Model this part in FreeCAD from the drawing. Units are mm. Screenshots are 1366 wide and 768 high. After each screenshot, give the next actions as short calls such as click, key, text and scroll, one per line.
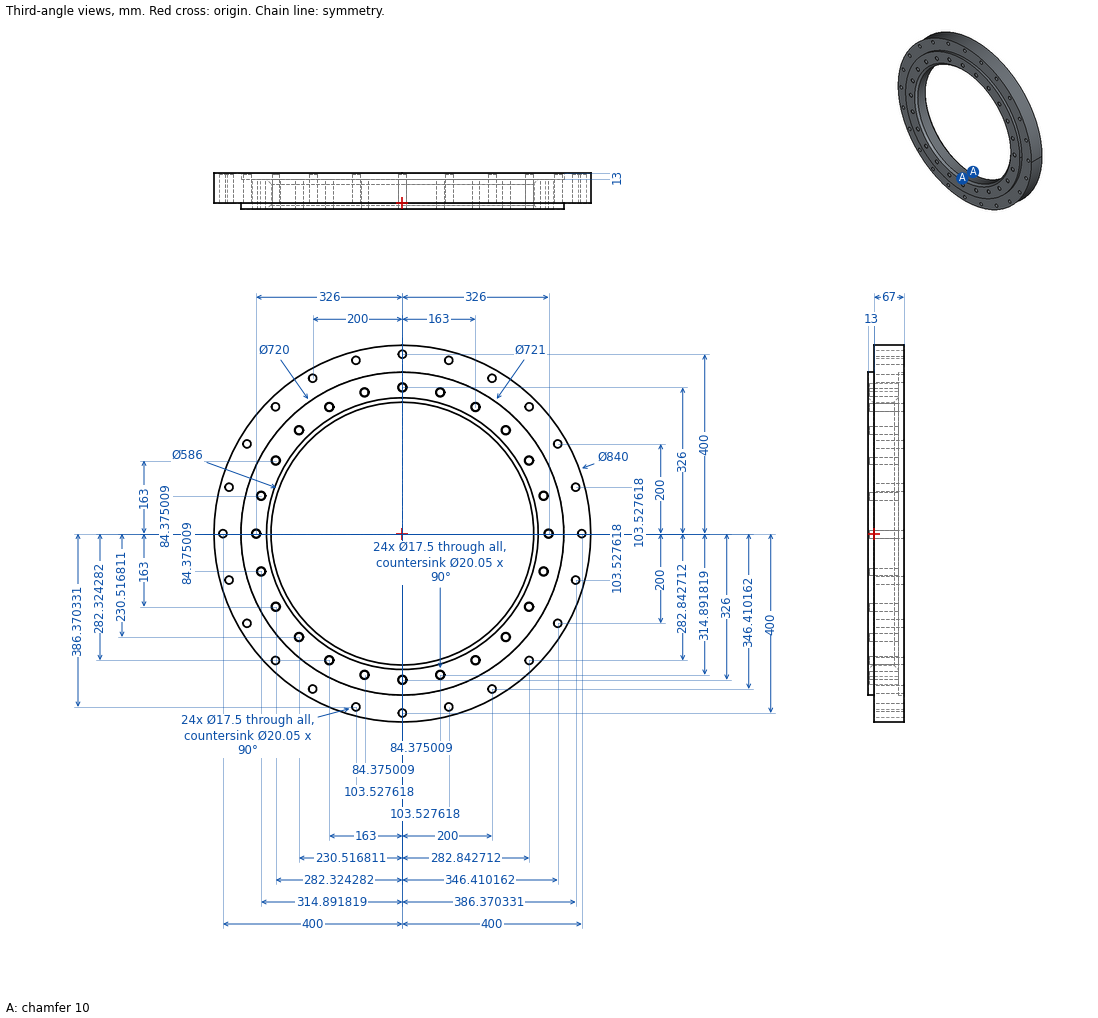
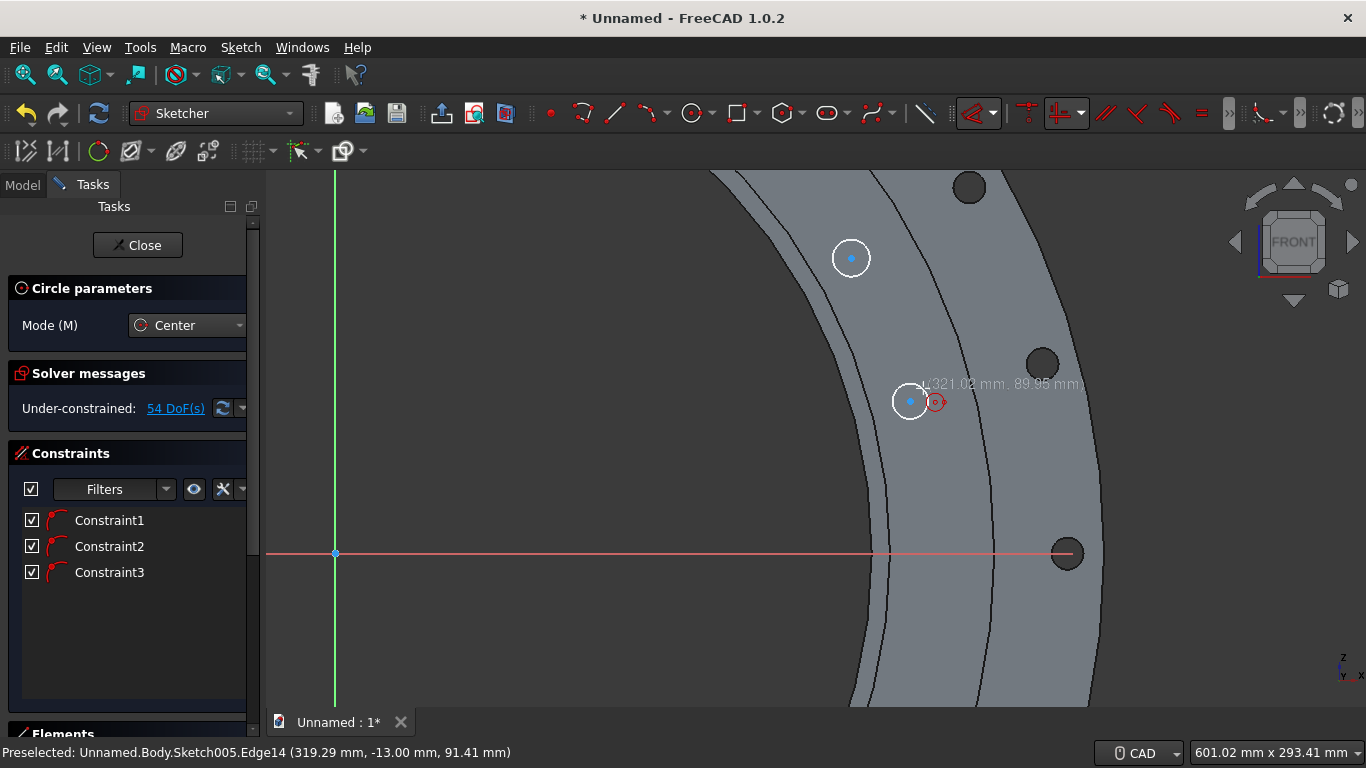
scroll(932, 554, up, 2)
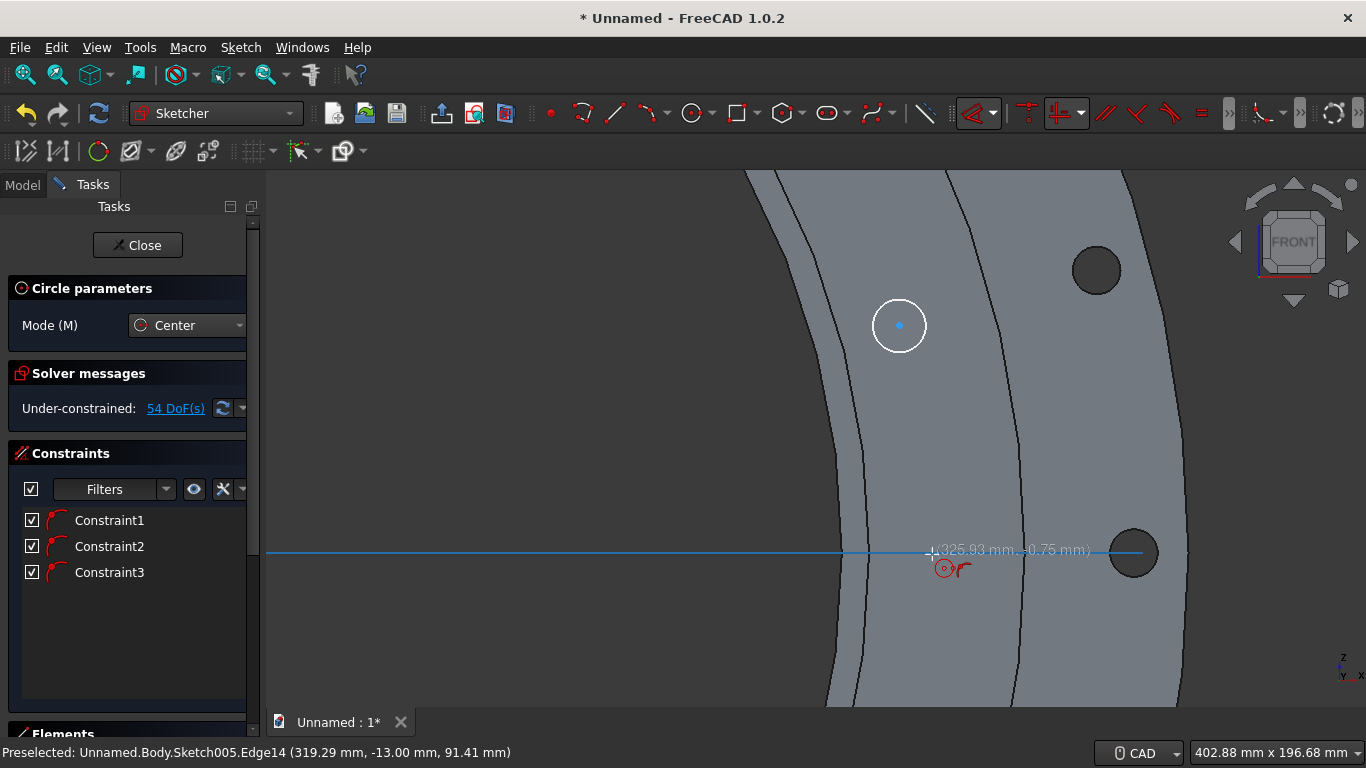
scroll(926, 410, down, 8)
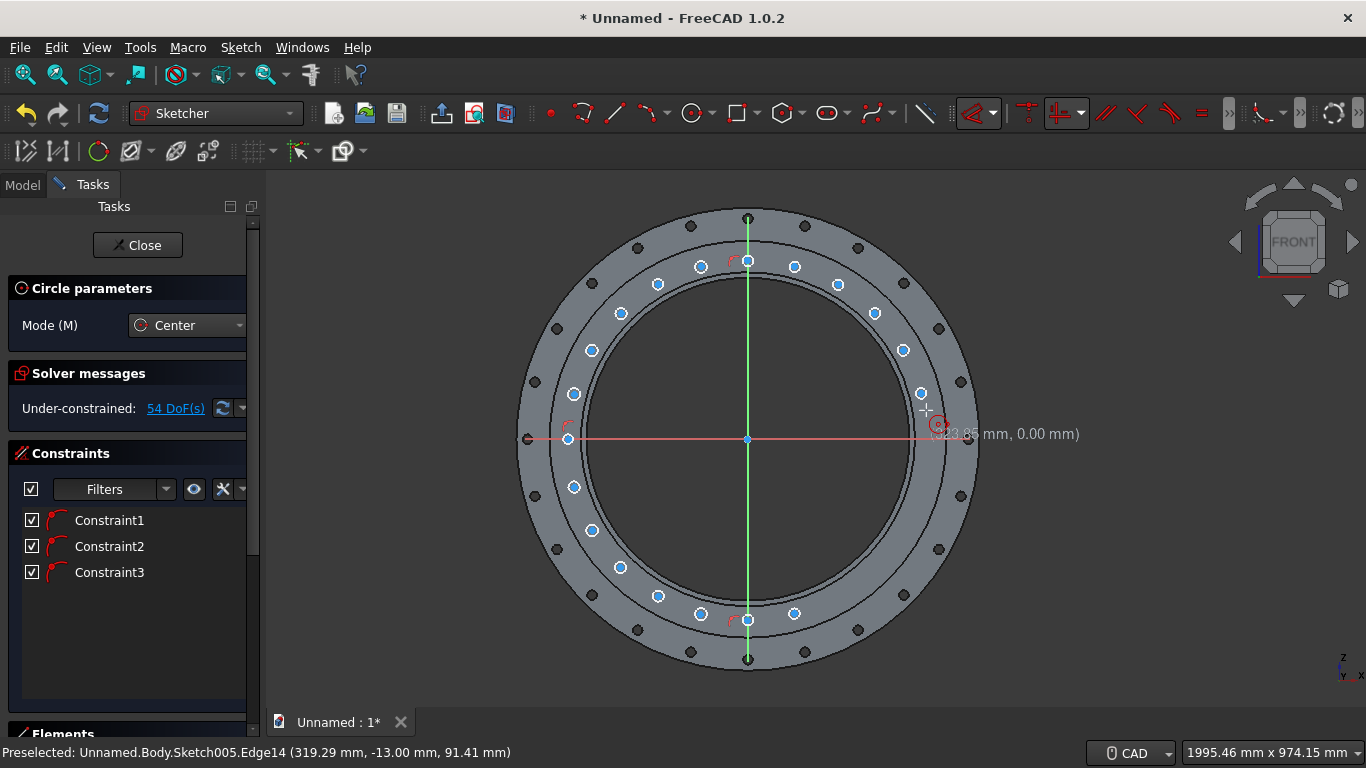
click(928, 439)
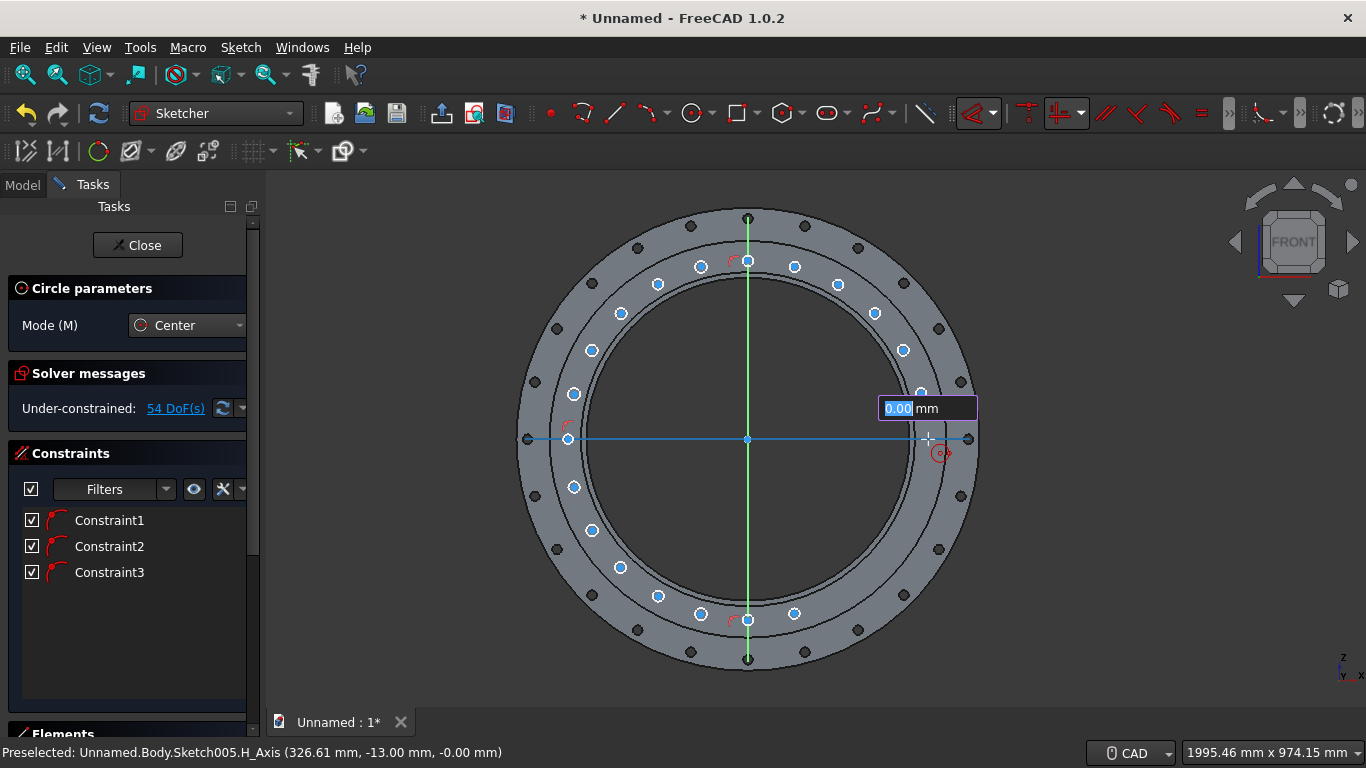
scroll(929, 435, up, 7)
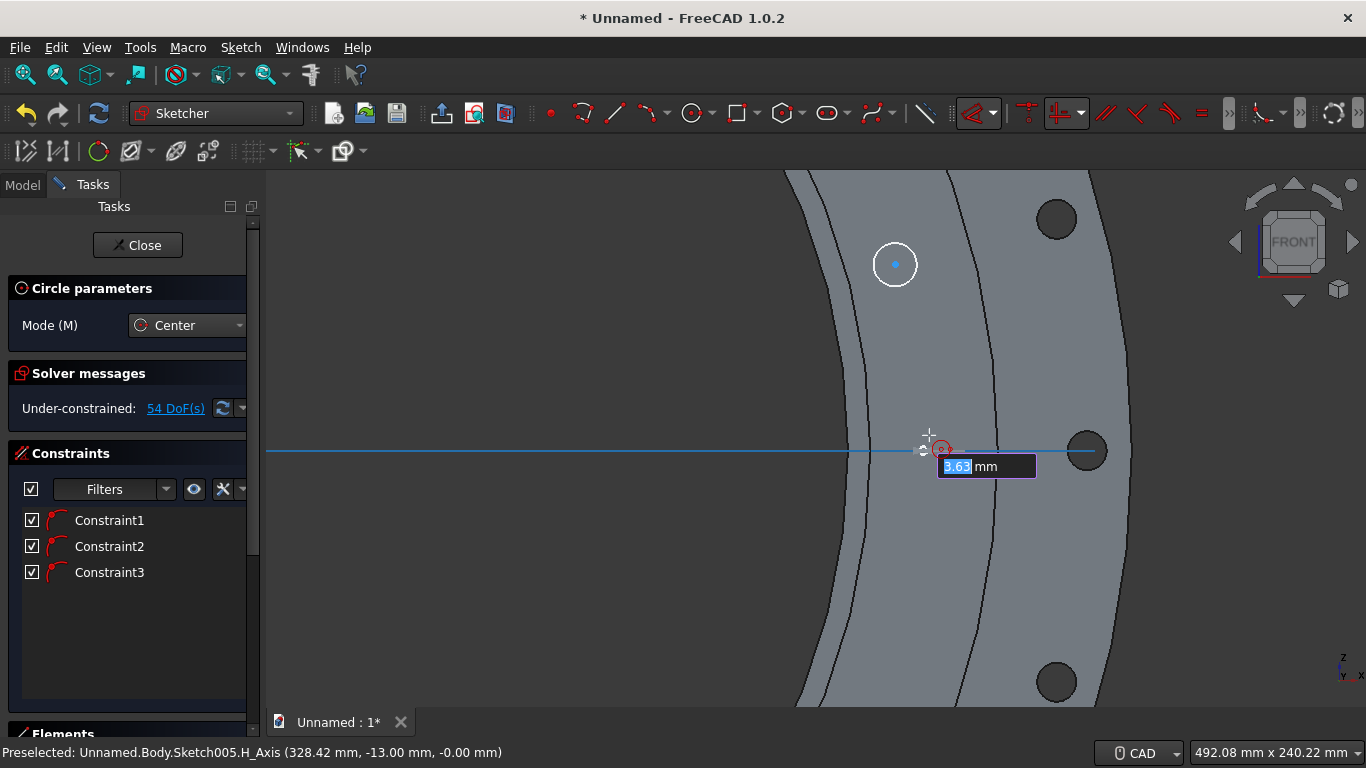
click(928, 432)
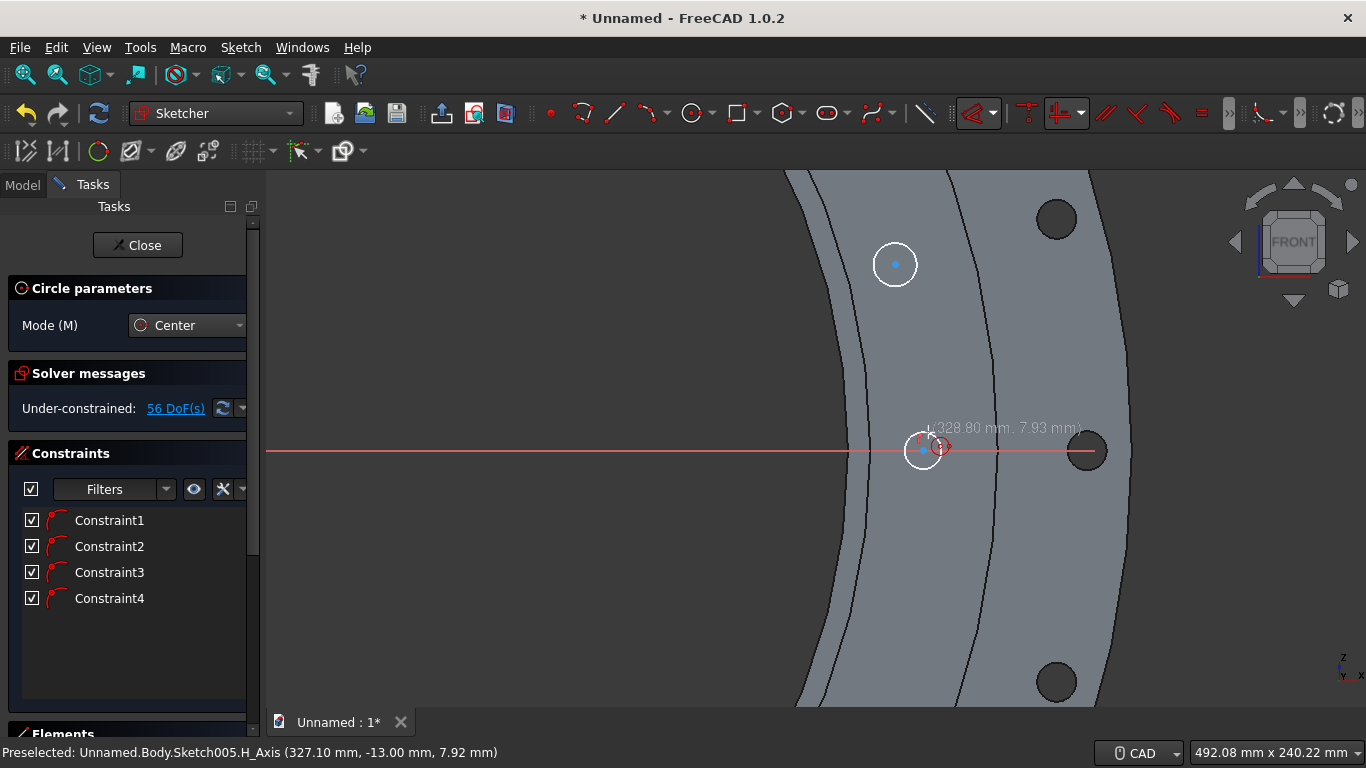
scroll(929, 435, down, 7)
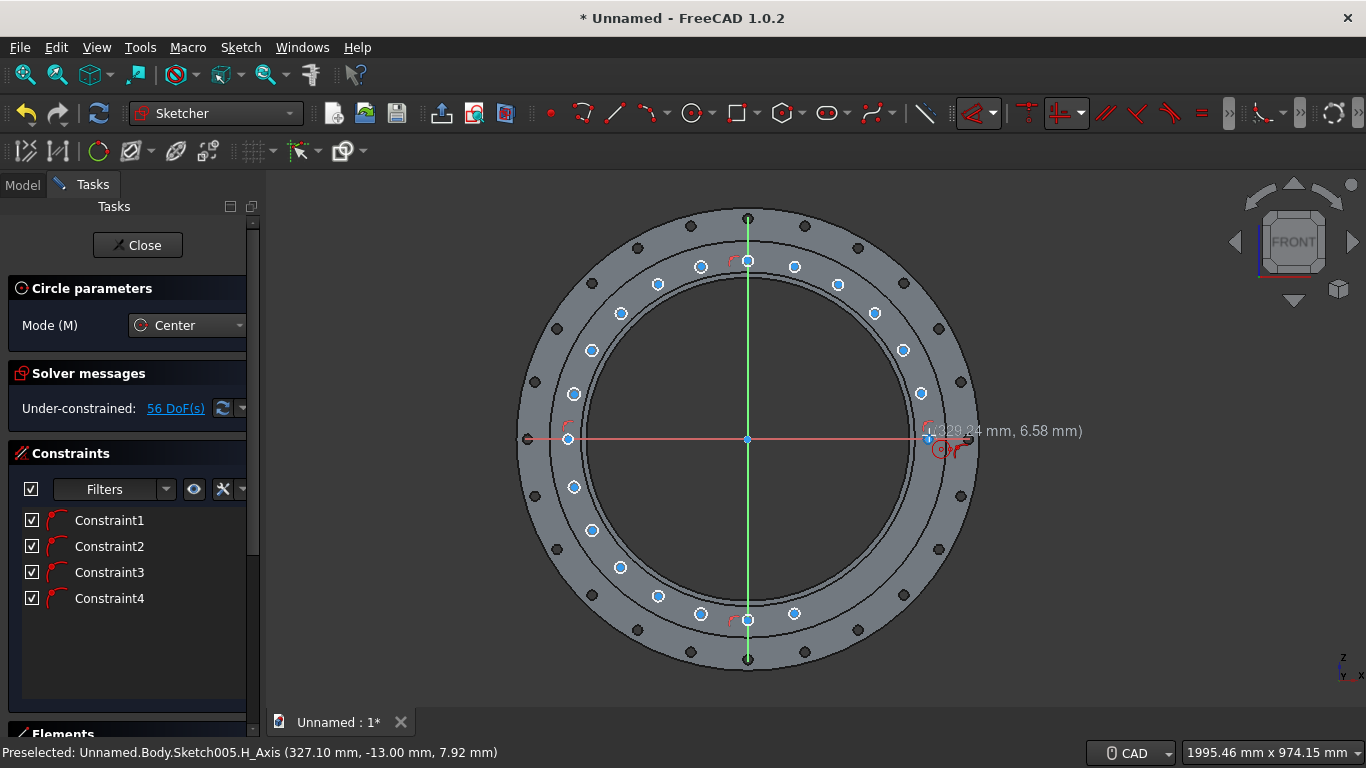
click(922, 486)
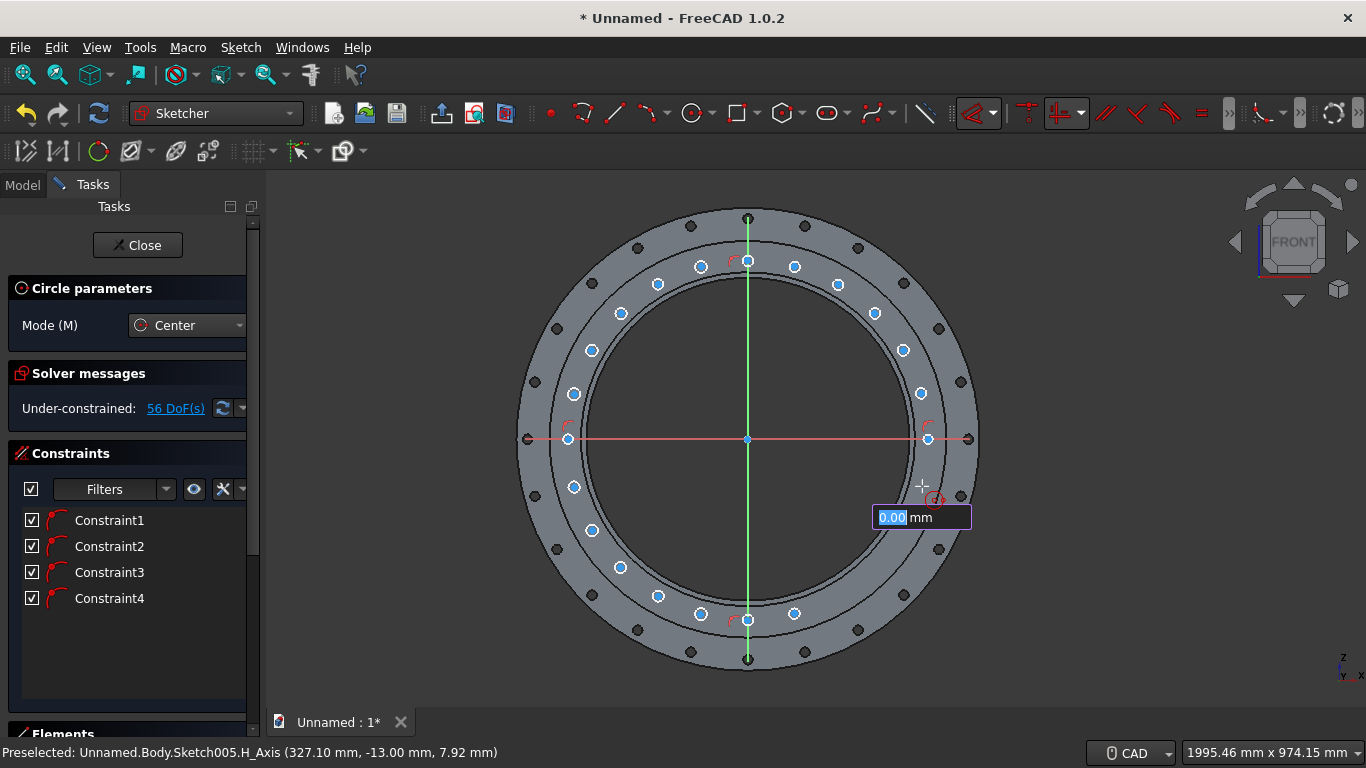
scroll(925, 482, up, 6)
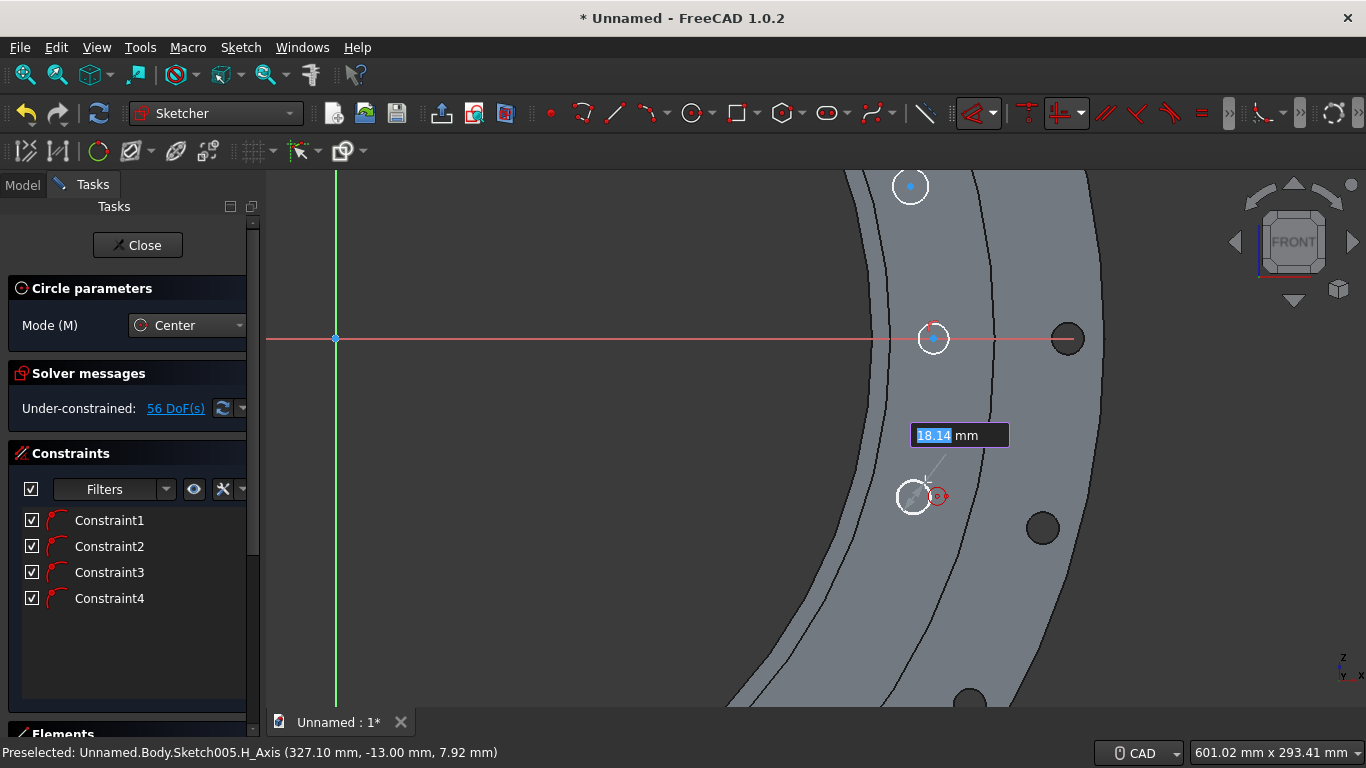
click(923, 482)